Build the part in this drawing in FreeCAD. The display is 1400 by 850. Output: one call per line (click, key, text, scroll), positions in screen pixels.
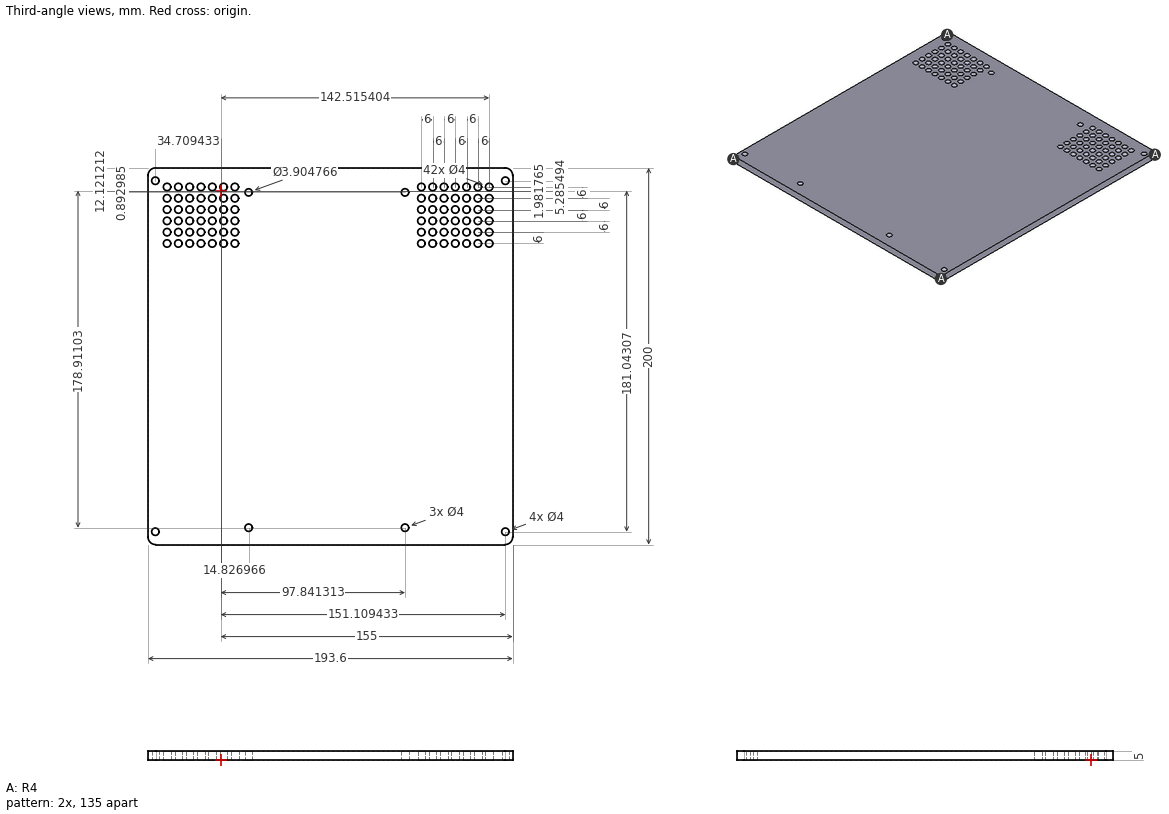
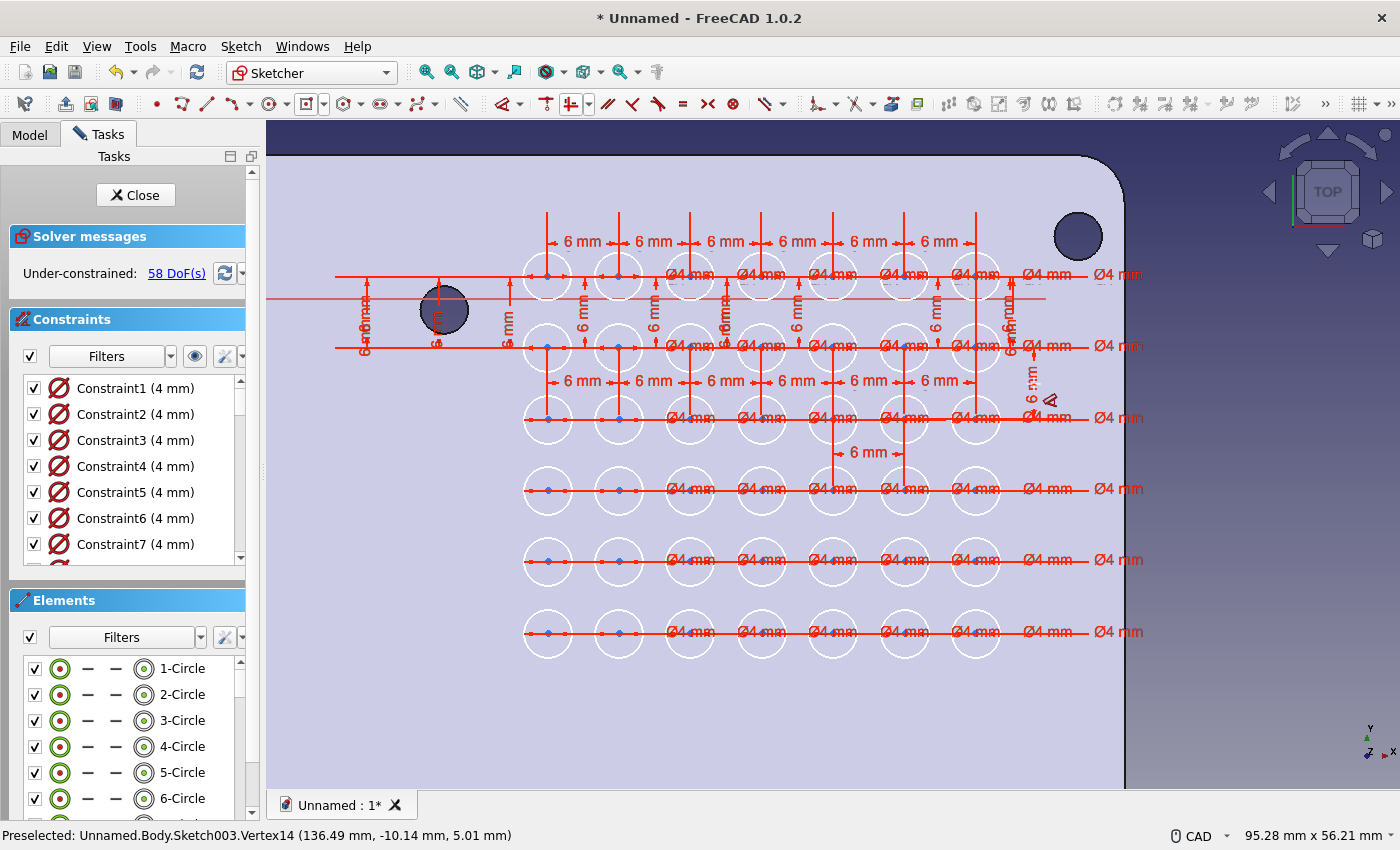
click(904, 419)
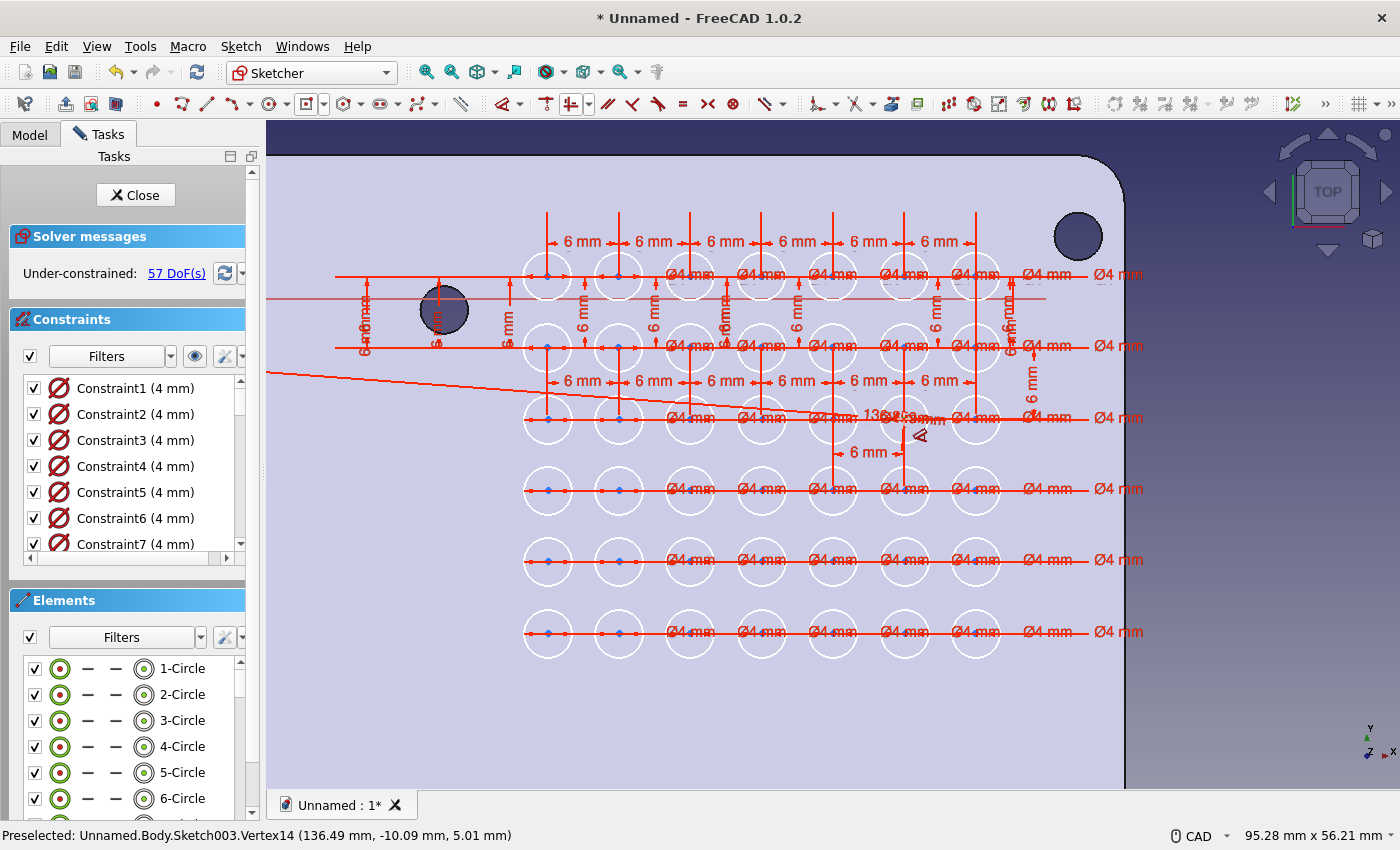
click(833, 420)
click(869, 361)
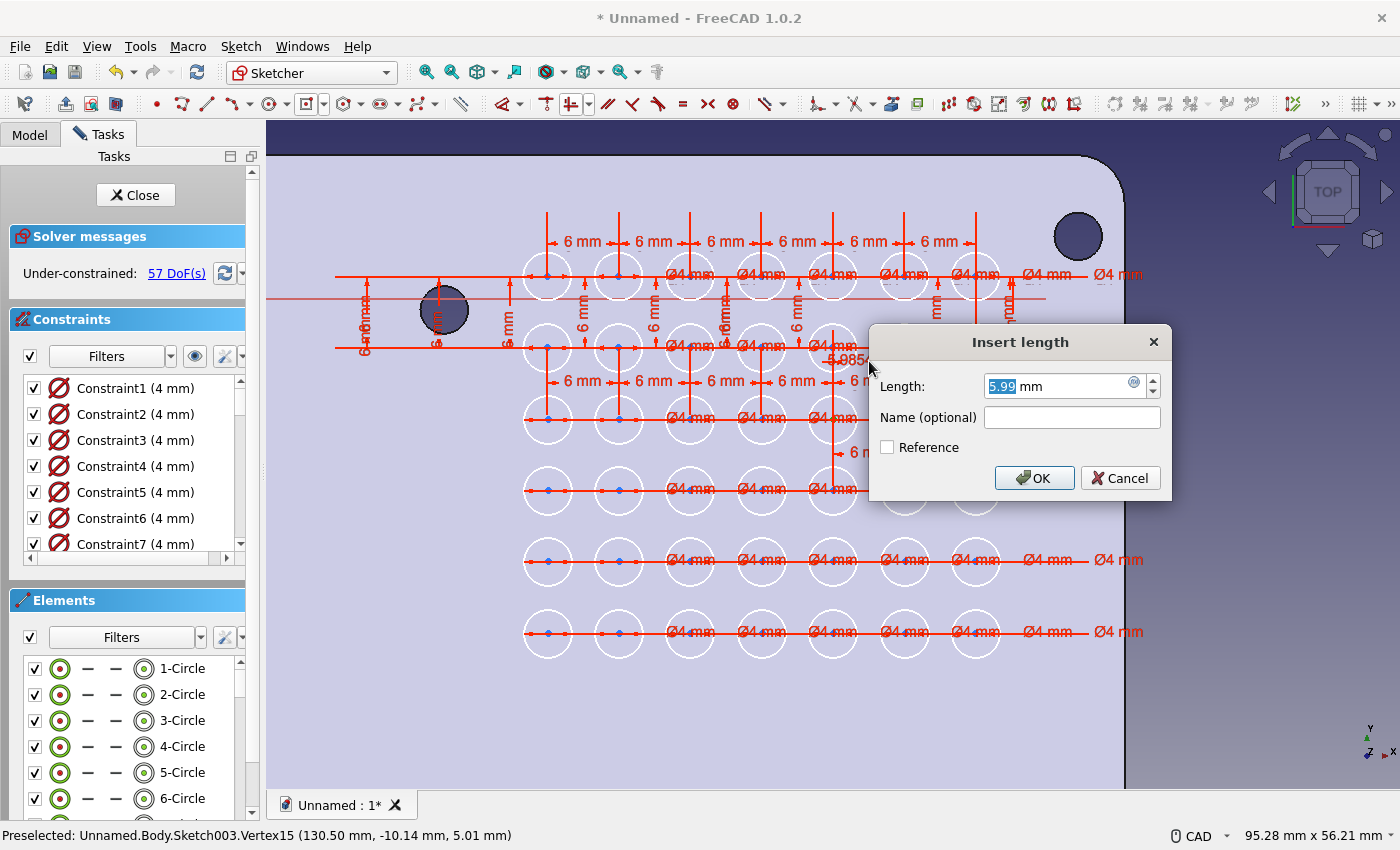
text(6)
key(Return)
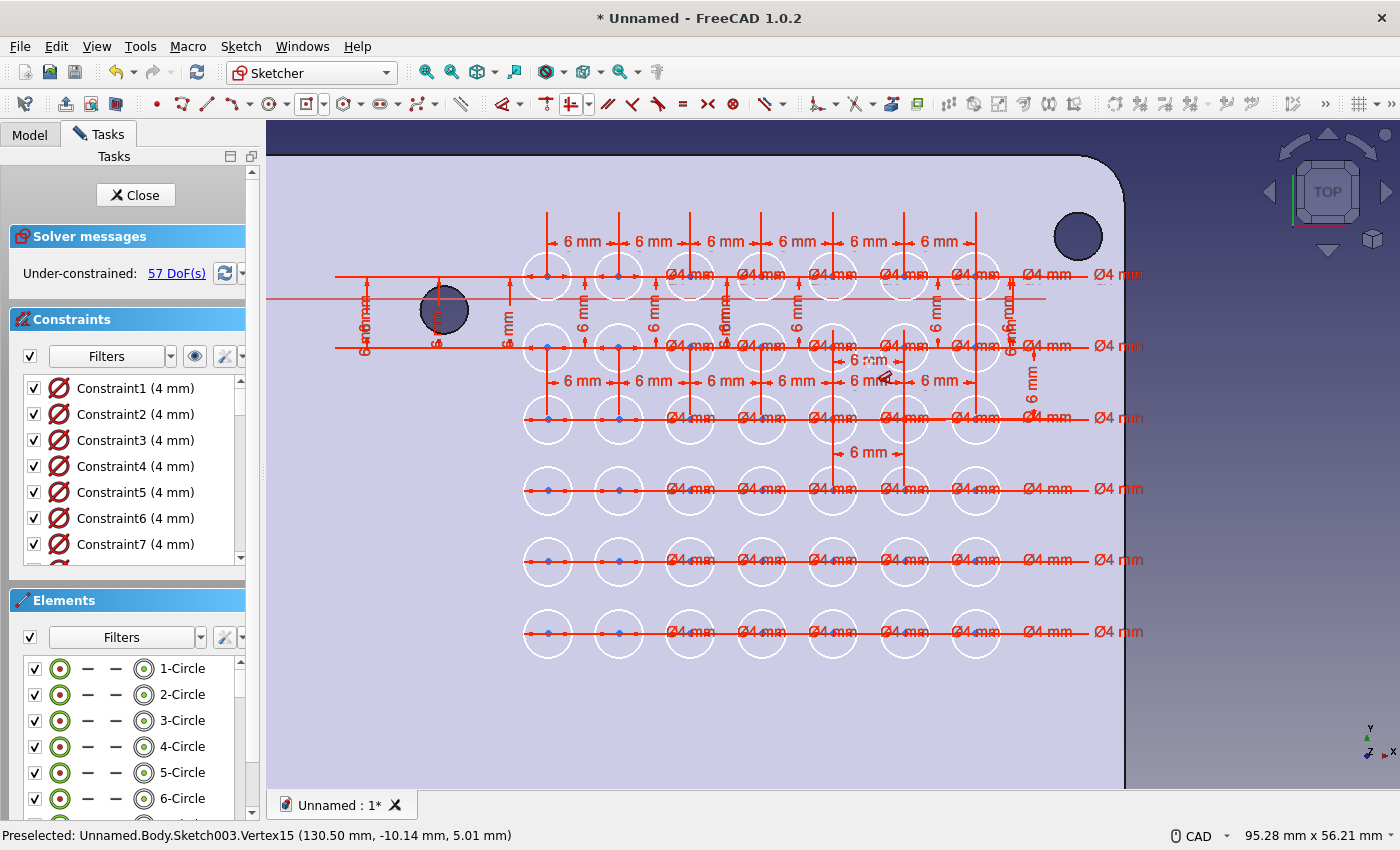
click(833, 348)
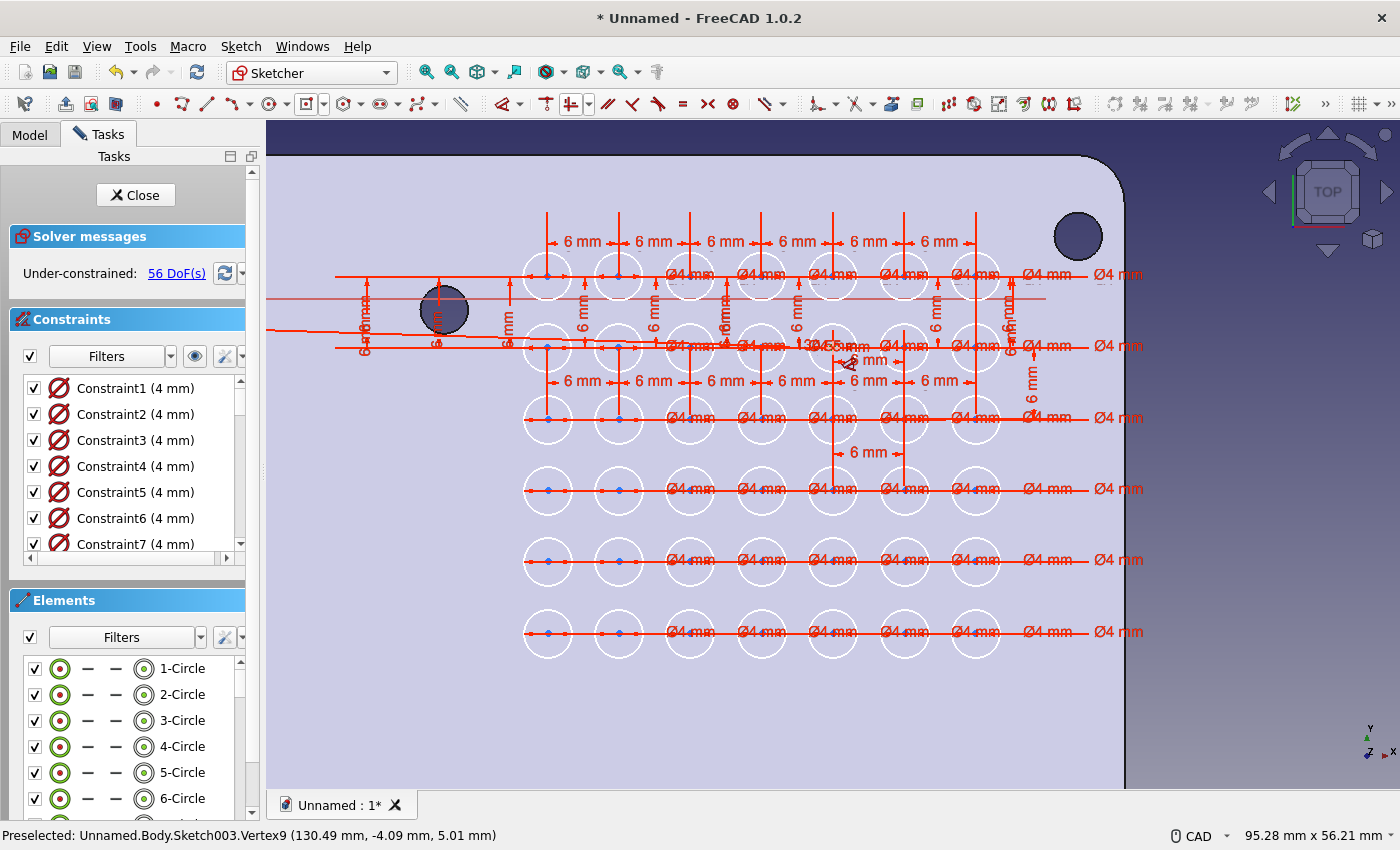
click(833, 420)
click(1013, 359)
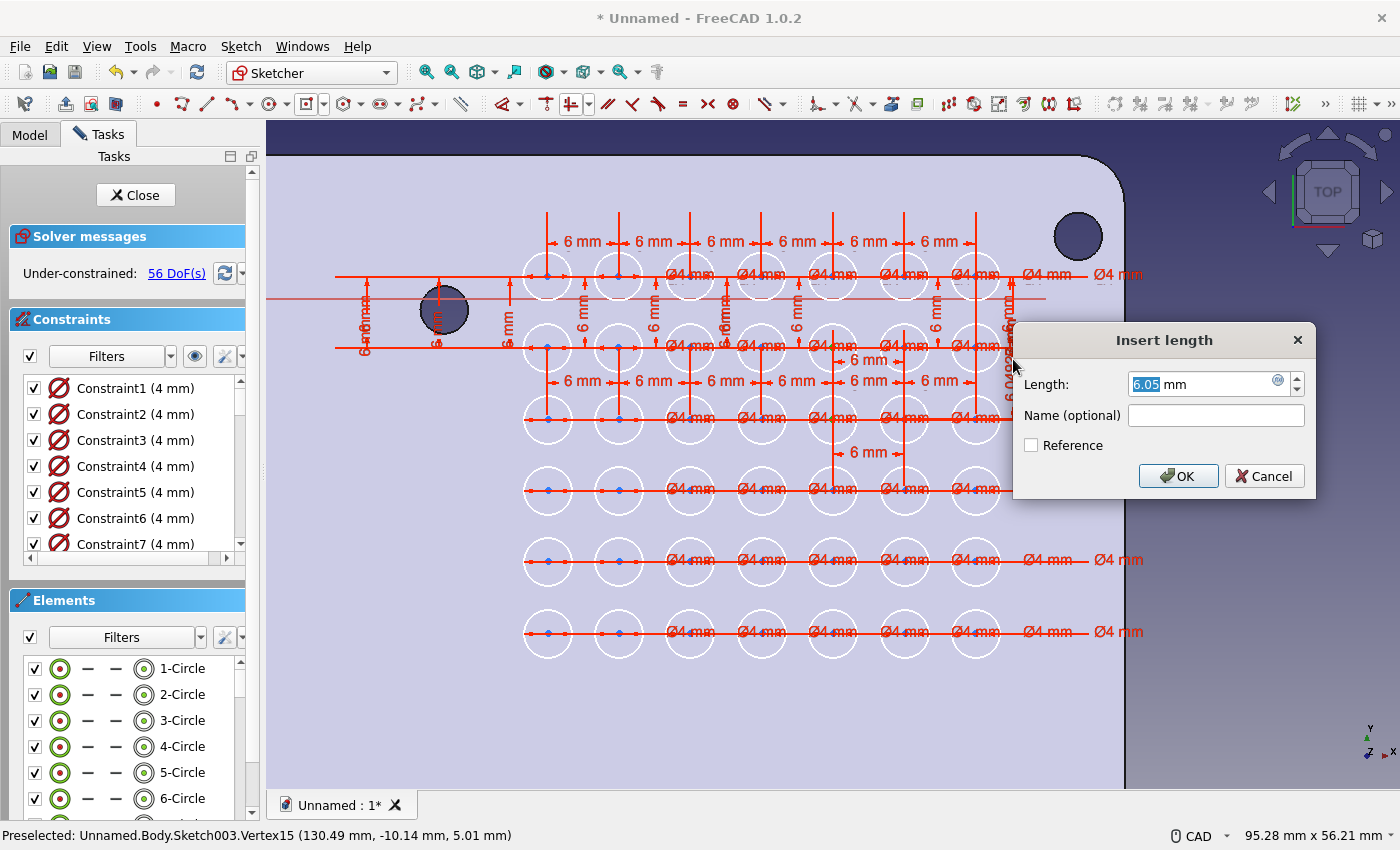
text(6)
key(Return)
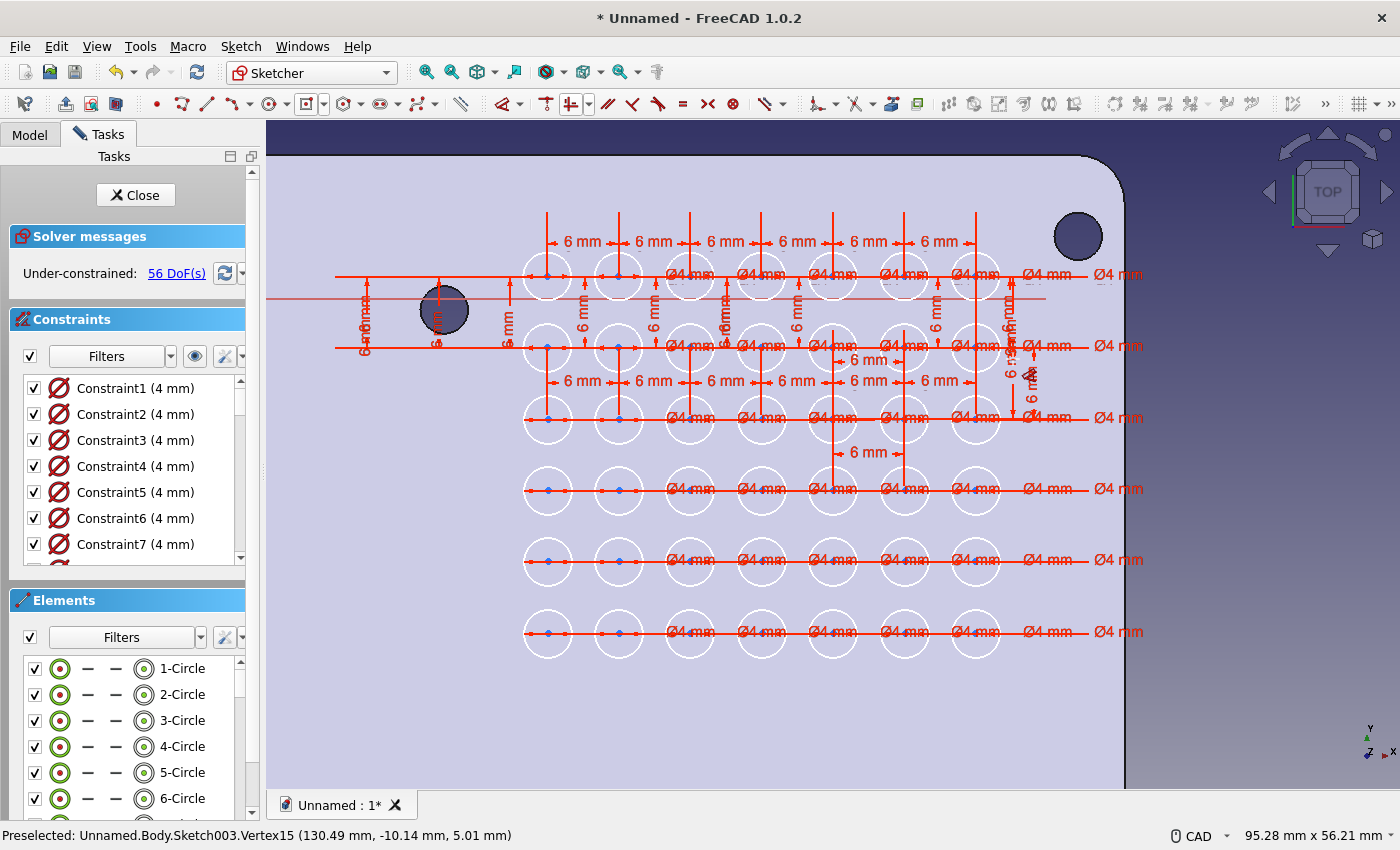
click(833, 419)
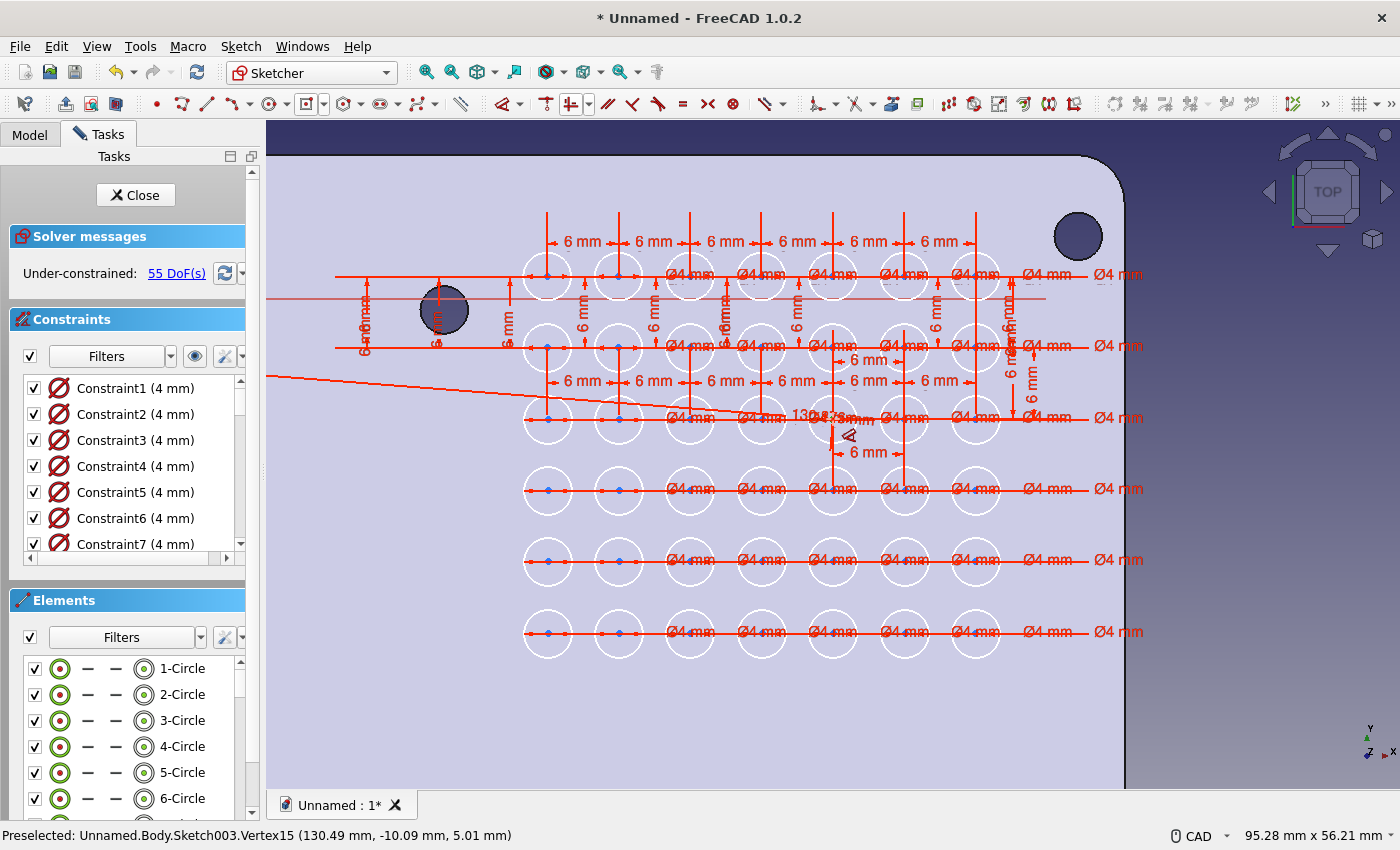
click(762, 420)
click(797, 454)